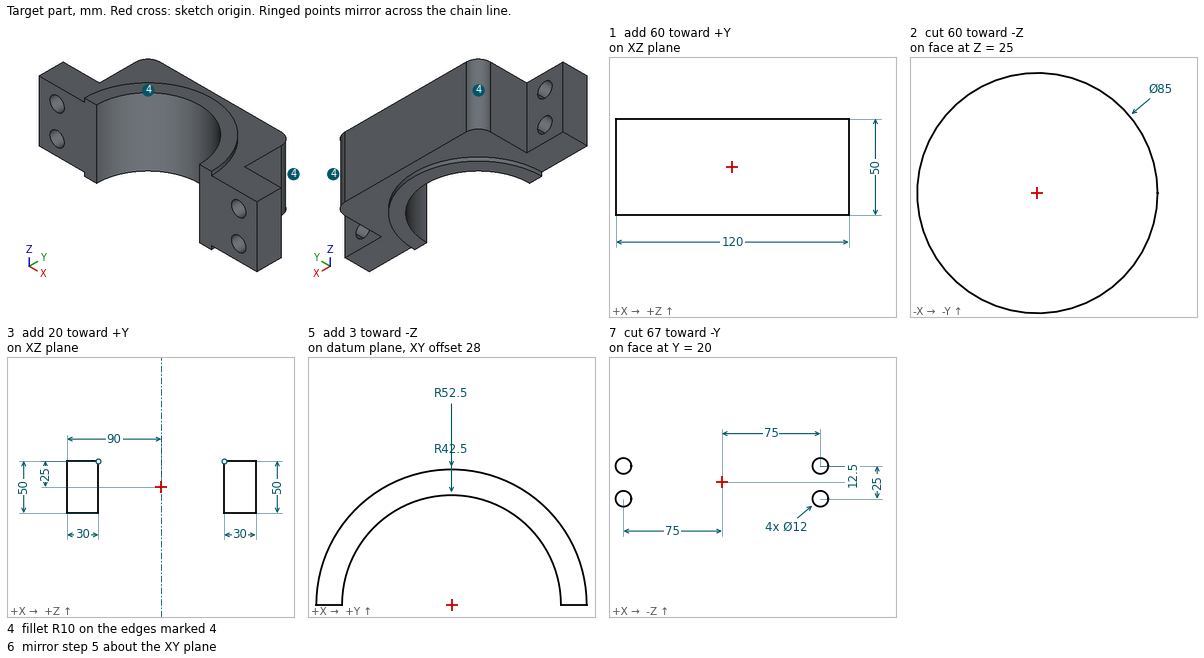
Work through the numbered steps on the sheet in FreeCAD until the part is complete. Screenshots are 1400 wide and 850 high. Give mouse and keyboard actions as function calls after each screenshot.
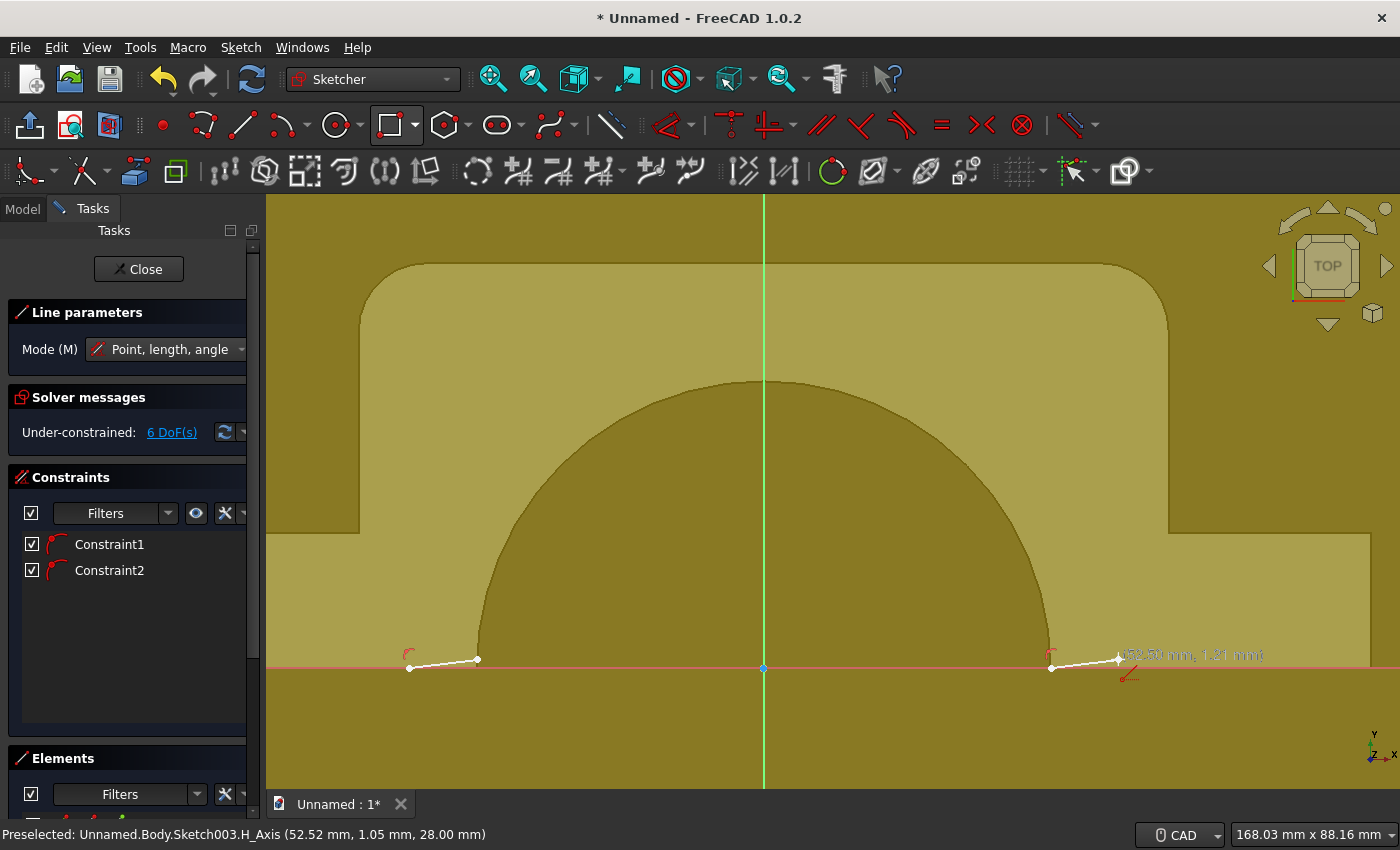
click(310, 126)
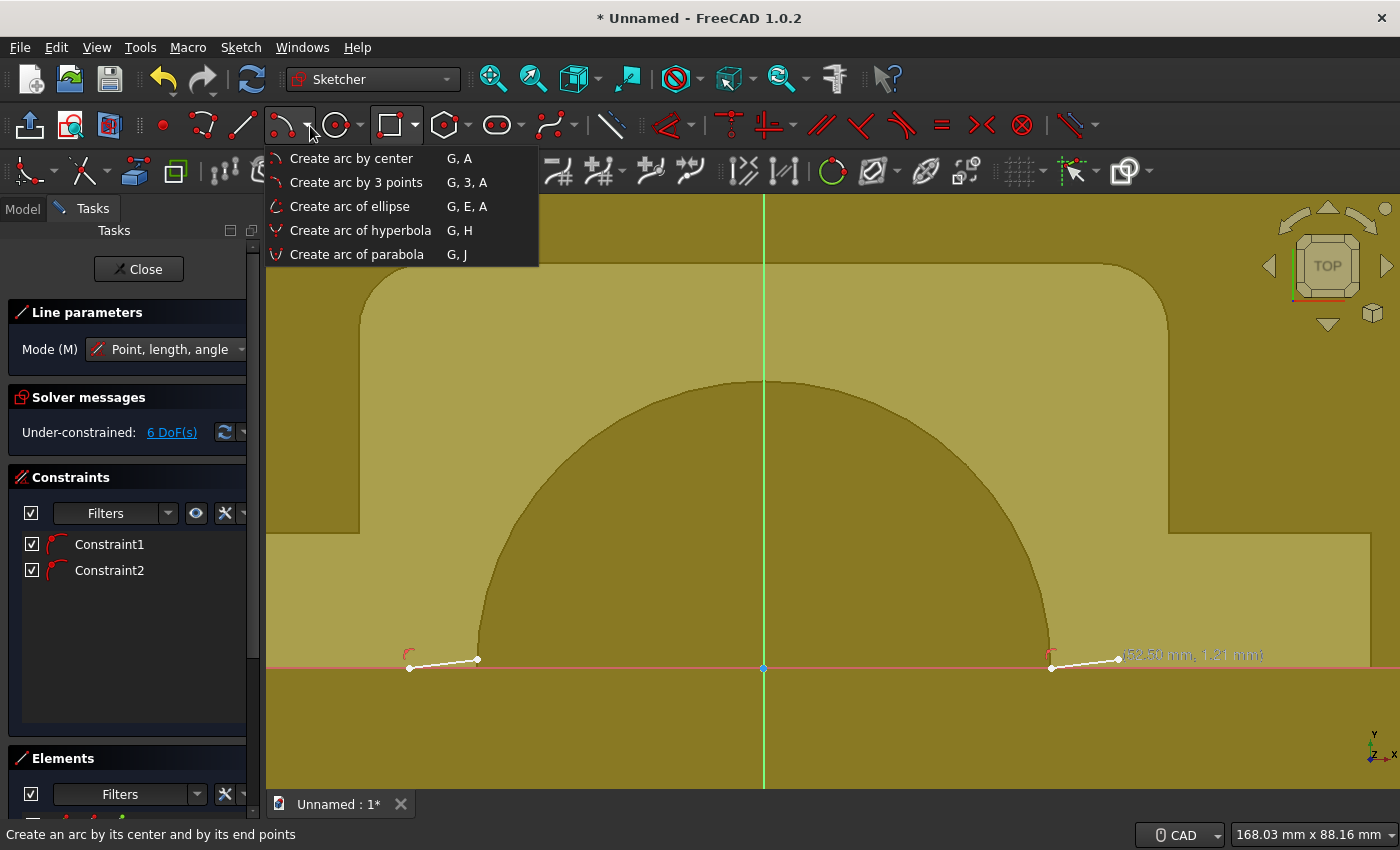
click(402, 182)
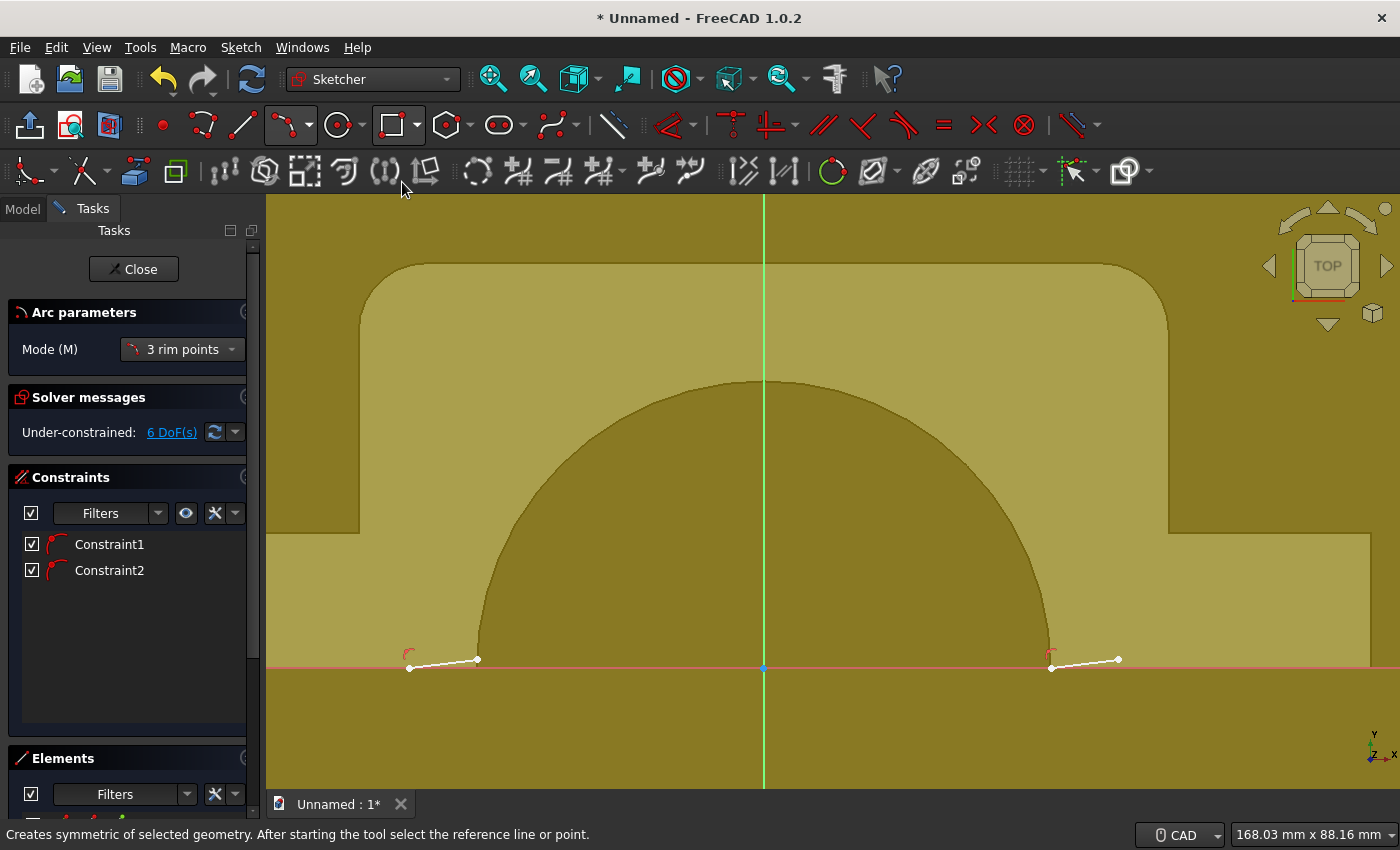
click(477, 660)
click(1051, 668)
click(852, 395)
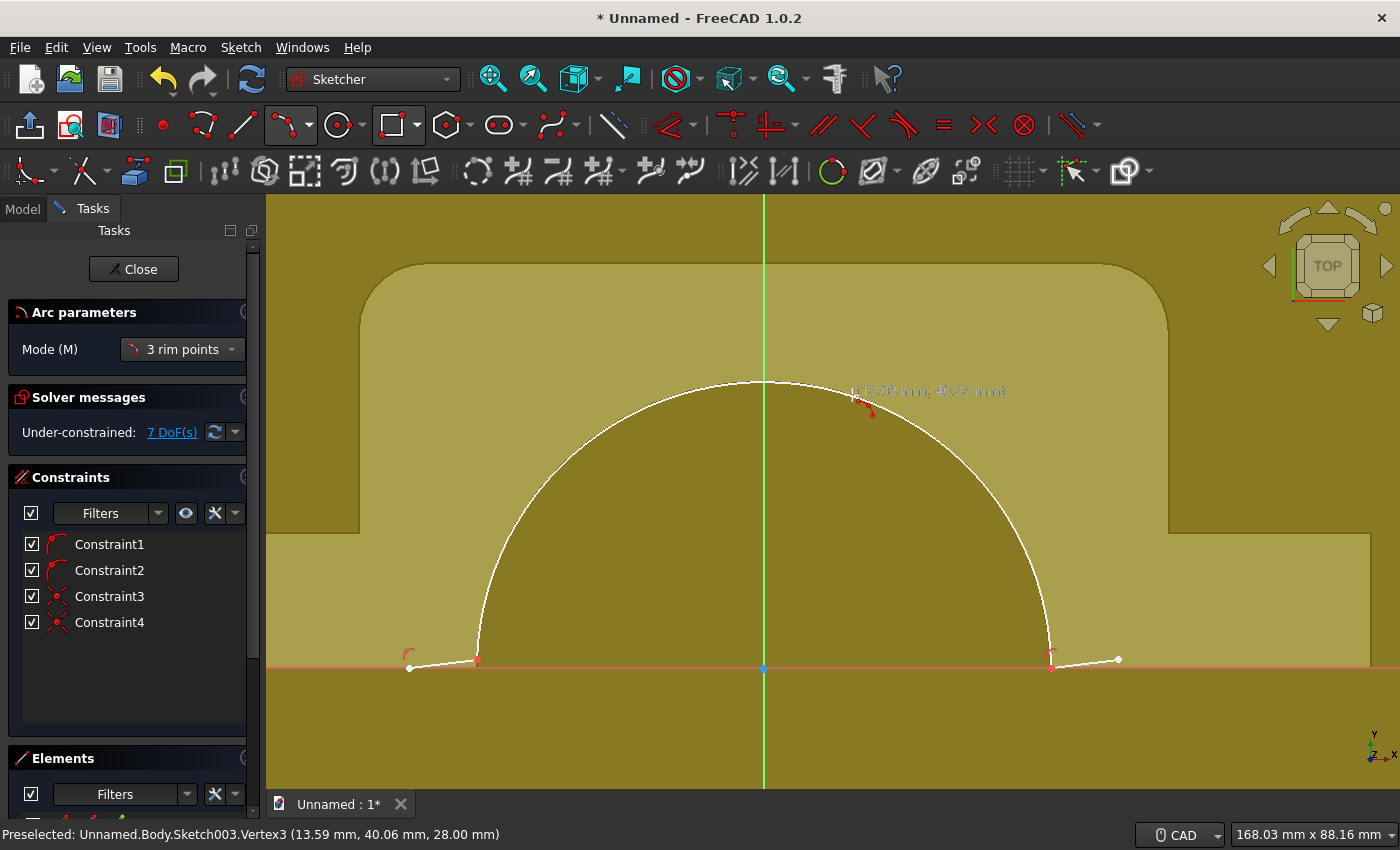
click(1118, 660)
click(409, 668)
click(873, 331)
key(Escape)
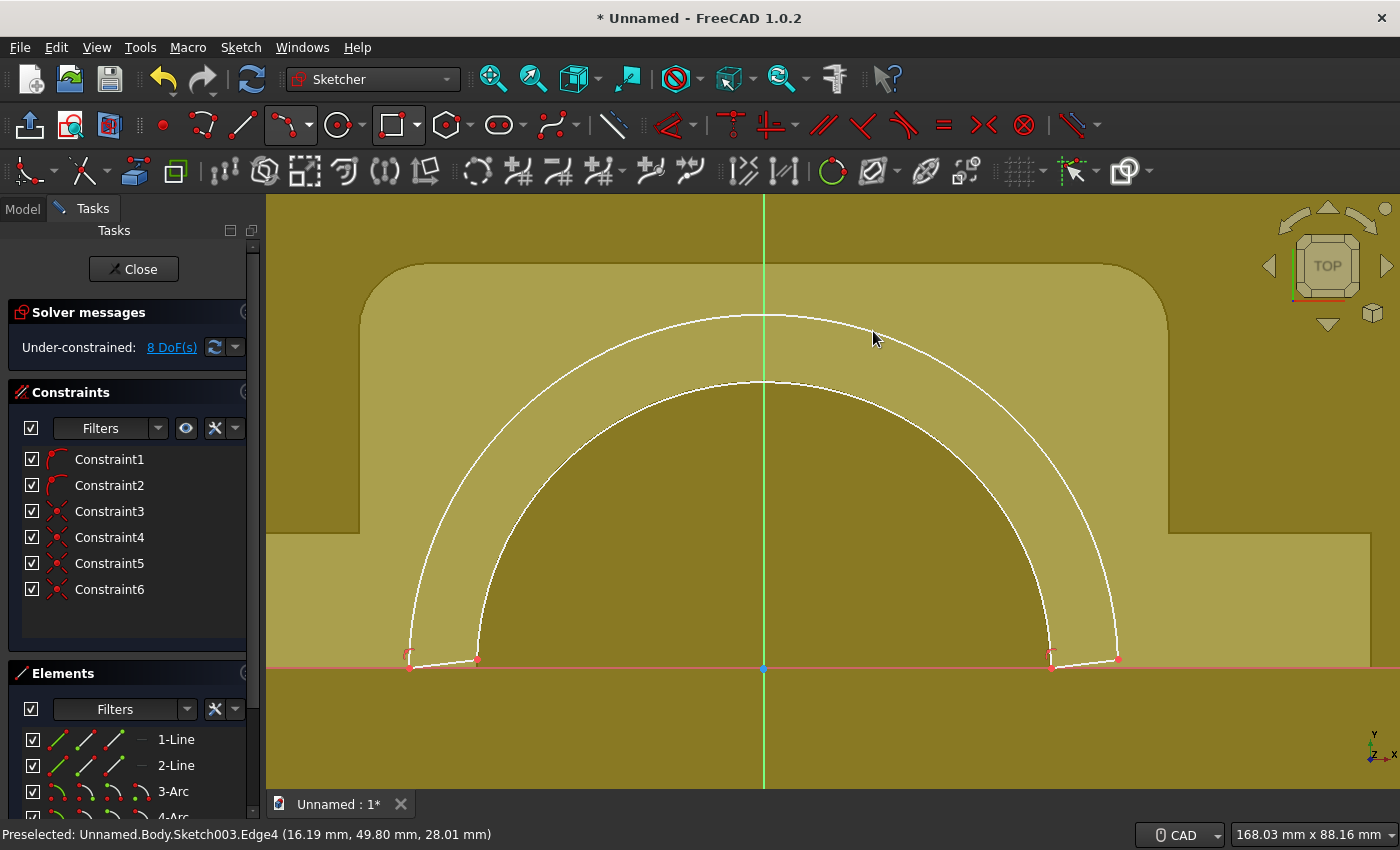
click(429, 666)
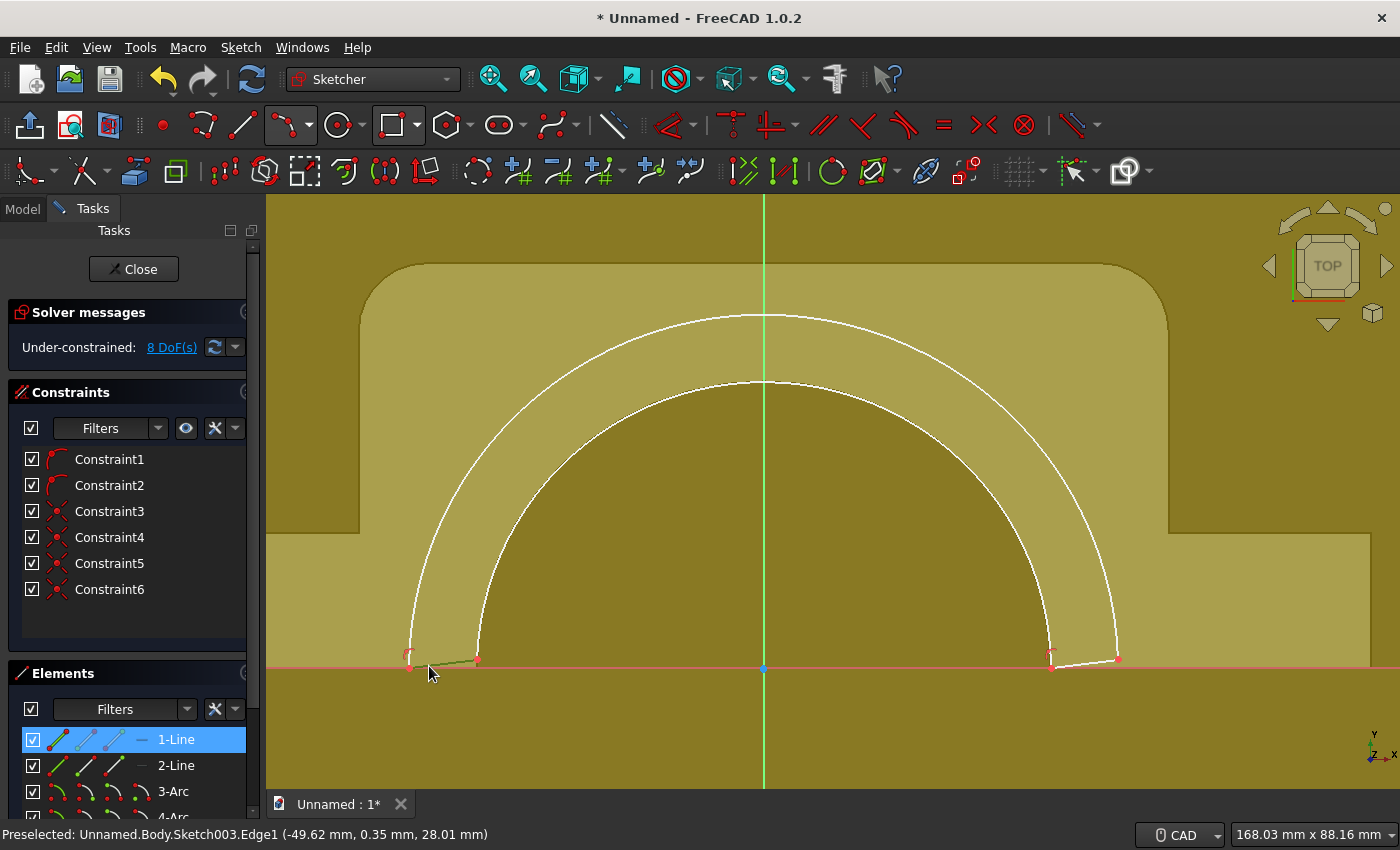
click(798, 126)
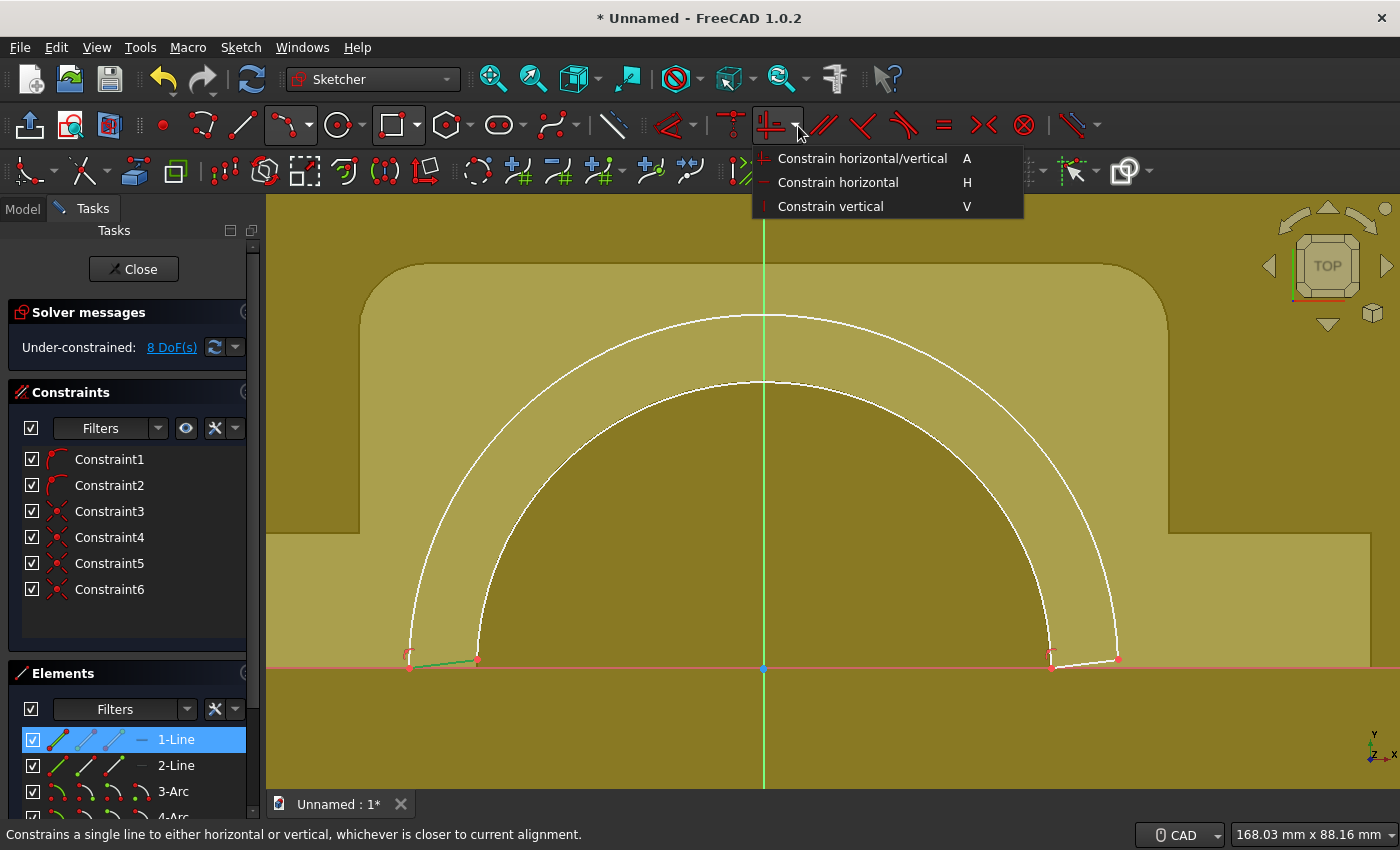
click(888, 182)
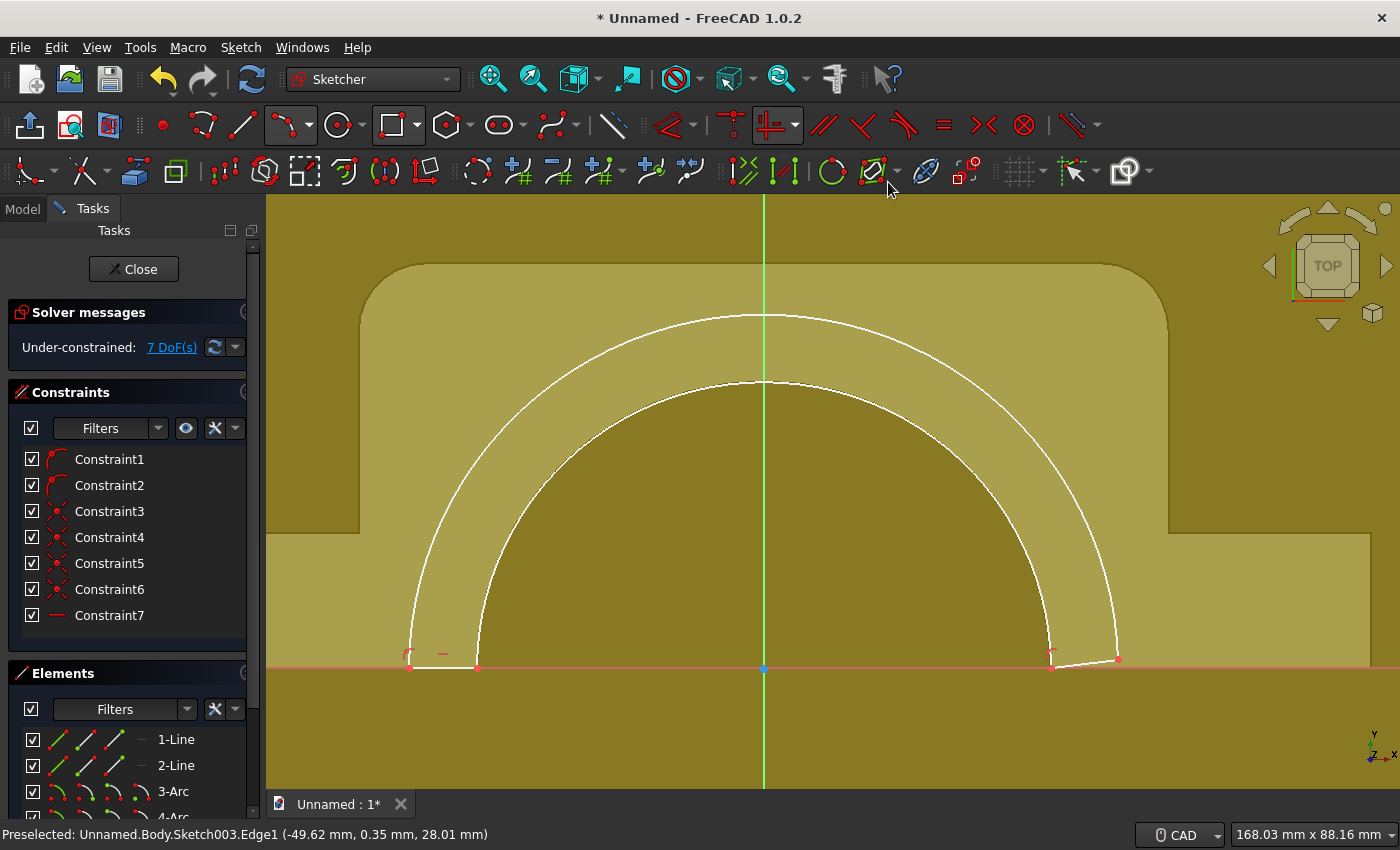
click(1071, 666)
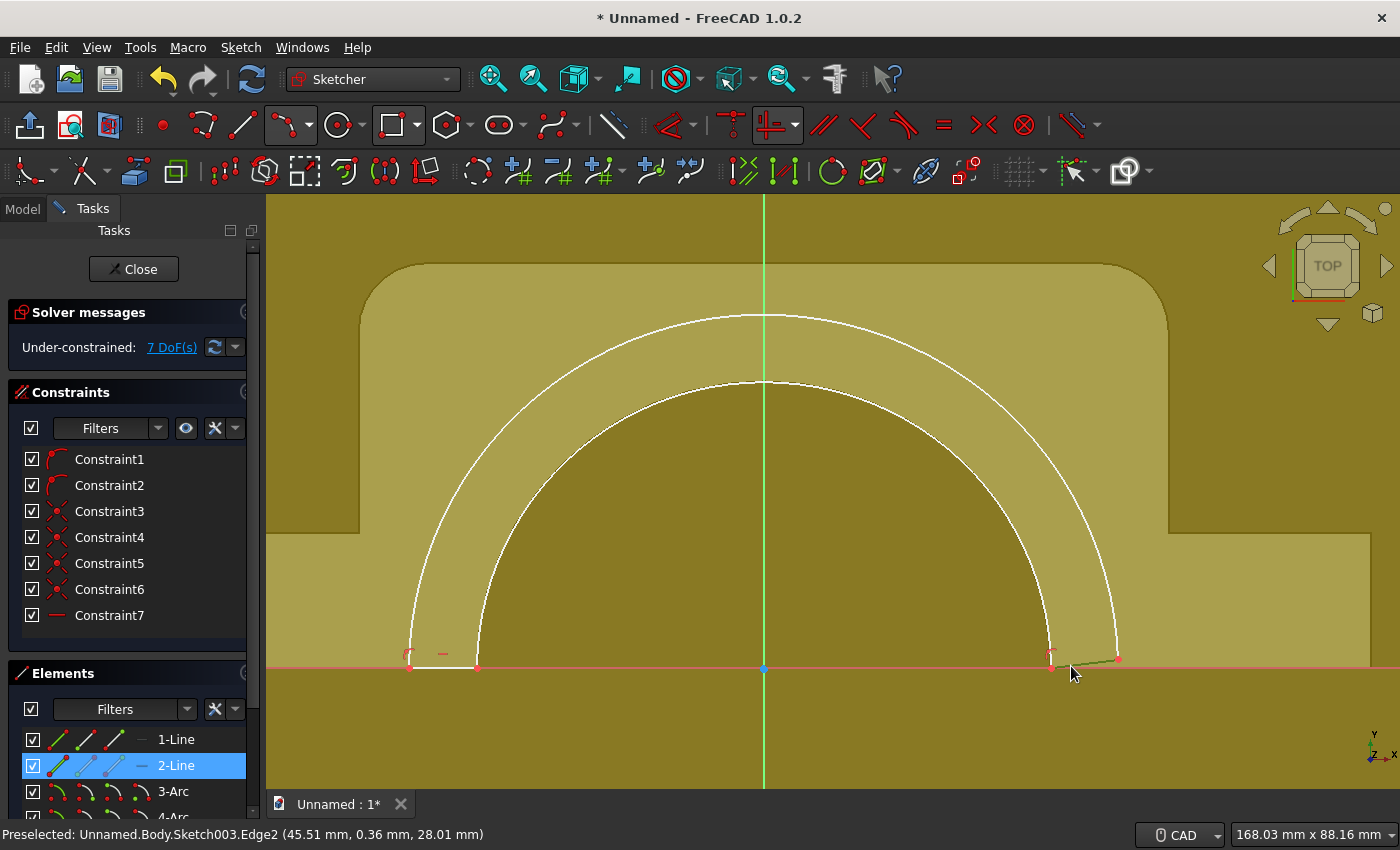
click(798, 126)